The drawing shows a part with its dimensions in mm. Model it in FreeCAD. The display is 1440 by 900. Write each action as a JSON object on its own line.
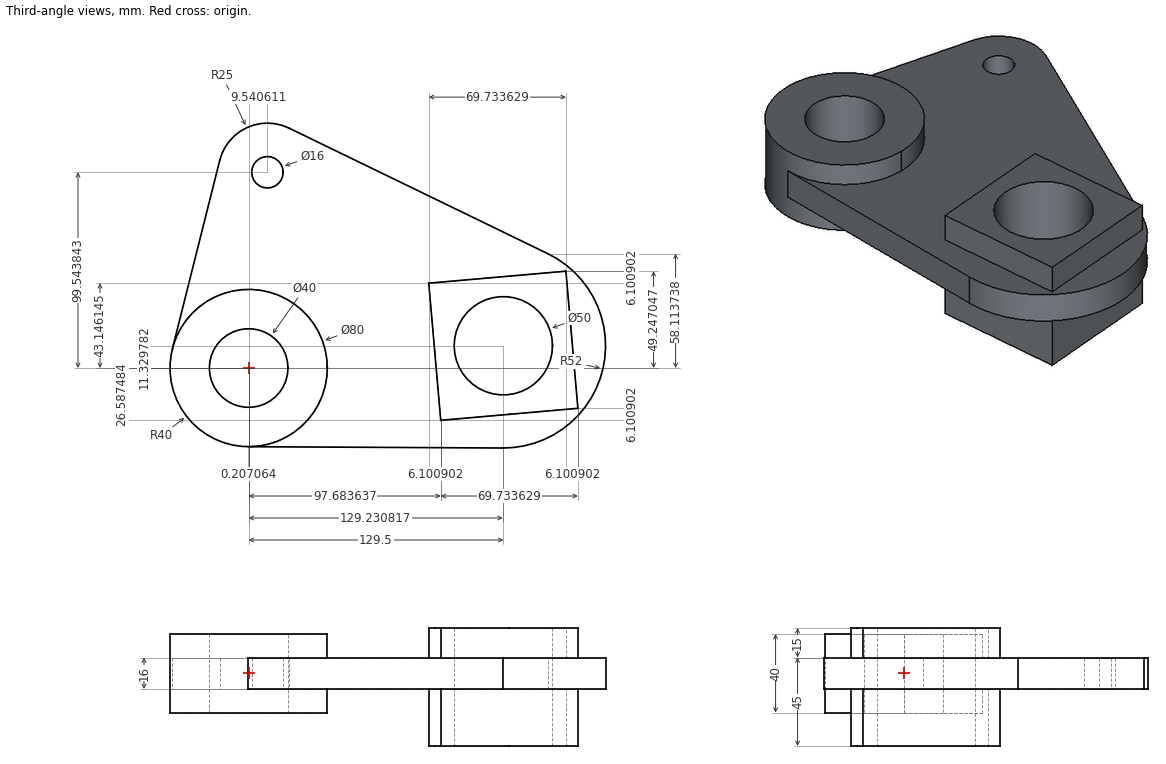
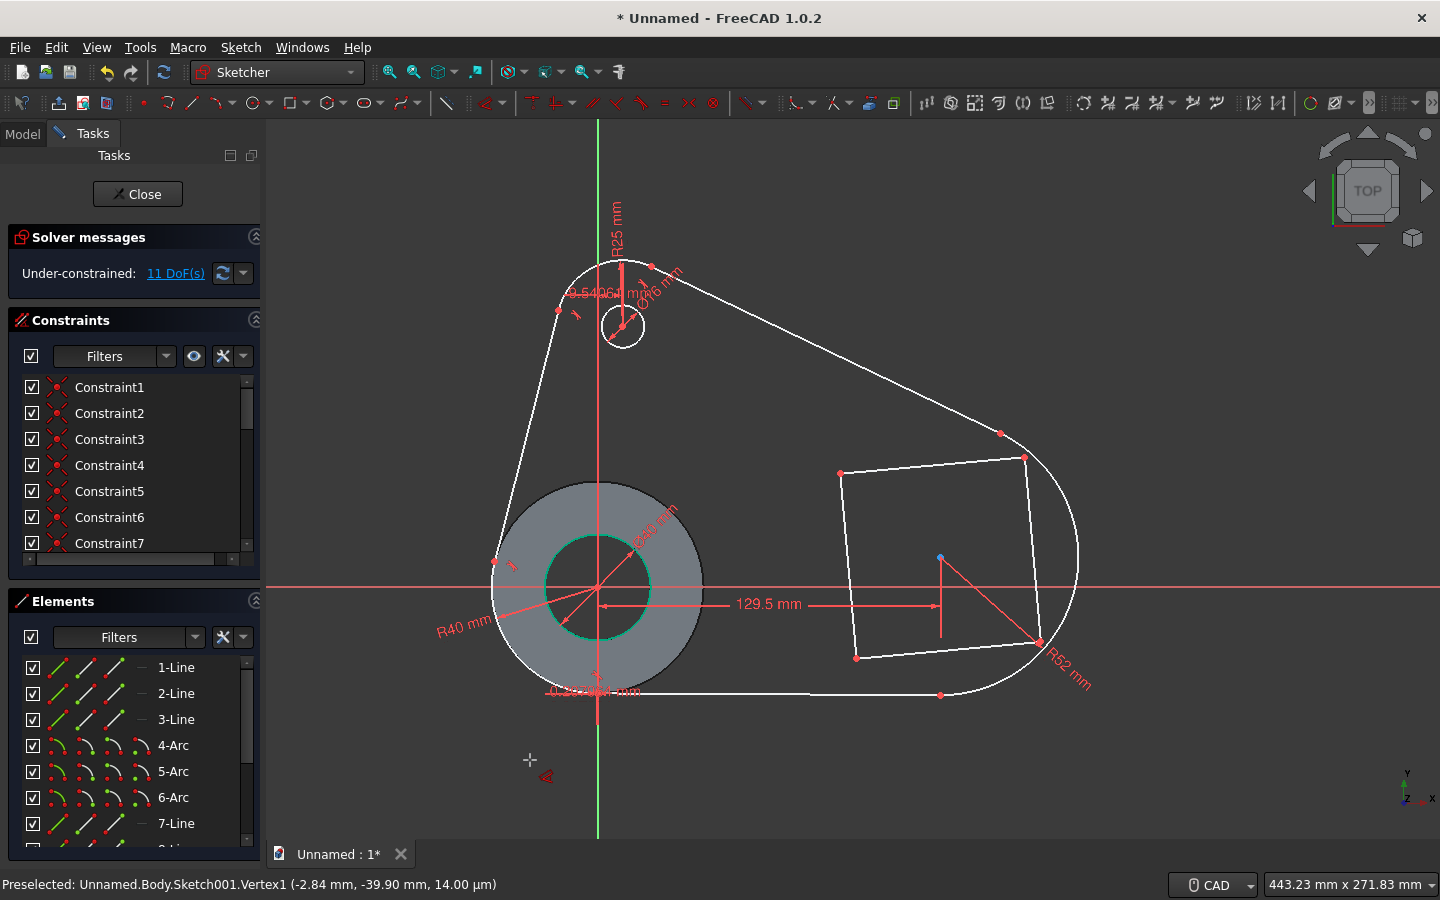
{"action": "scroll", "coordinate": [852, 603], "scroll_direction": "up", "scroll_amount": 5}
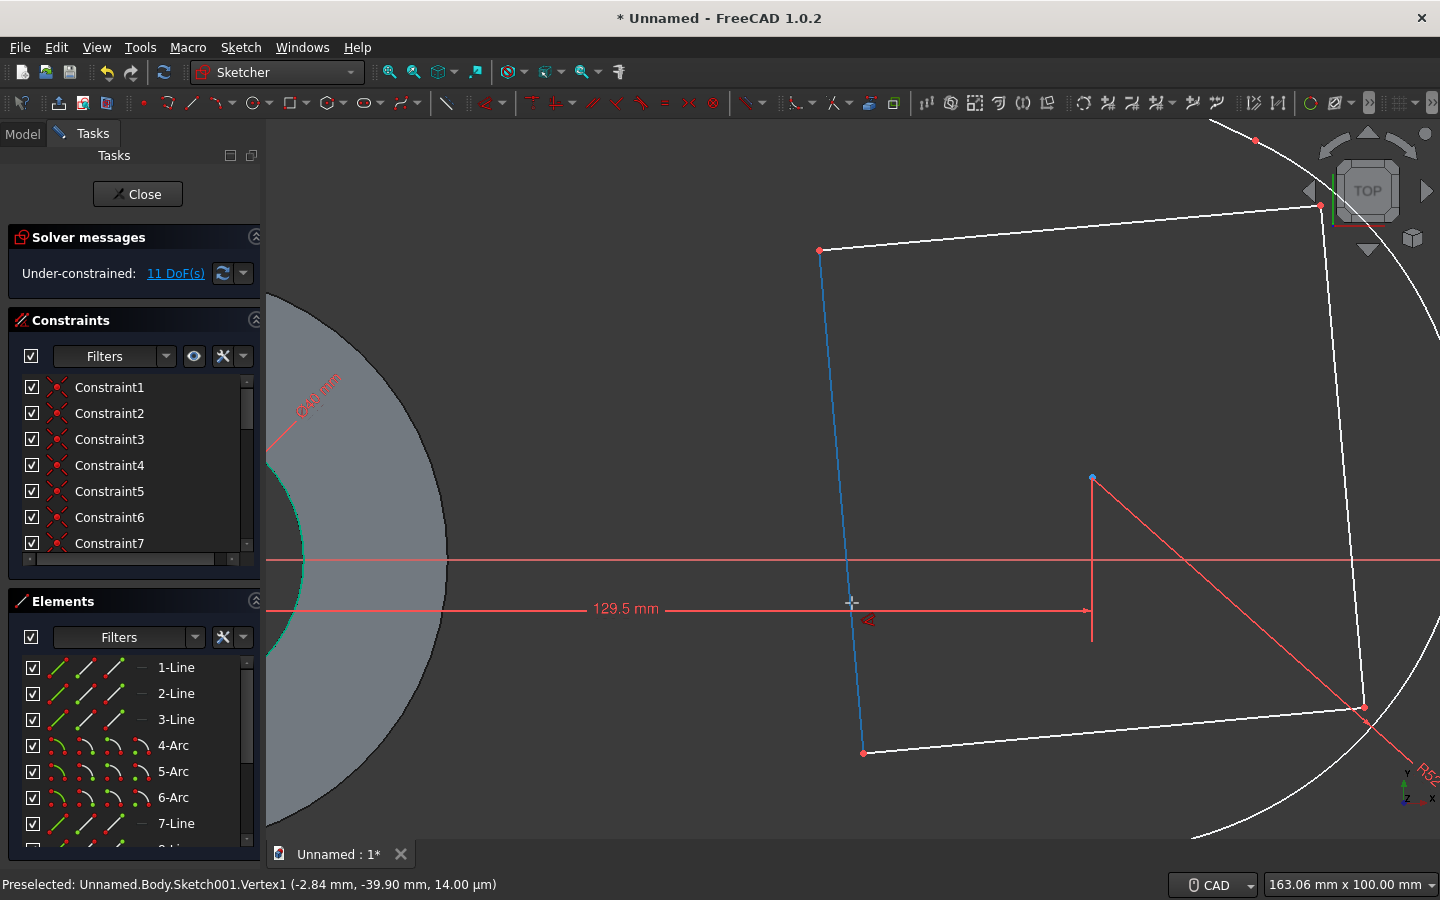
{"action": "left_click", "coordinate": [850, 603]}
{"action": "left_click", "coordinate": [841, 788]}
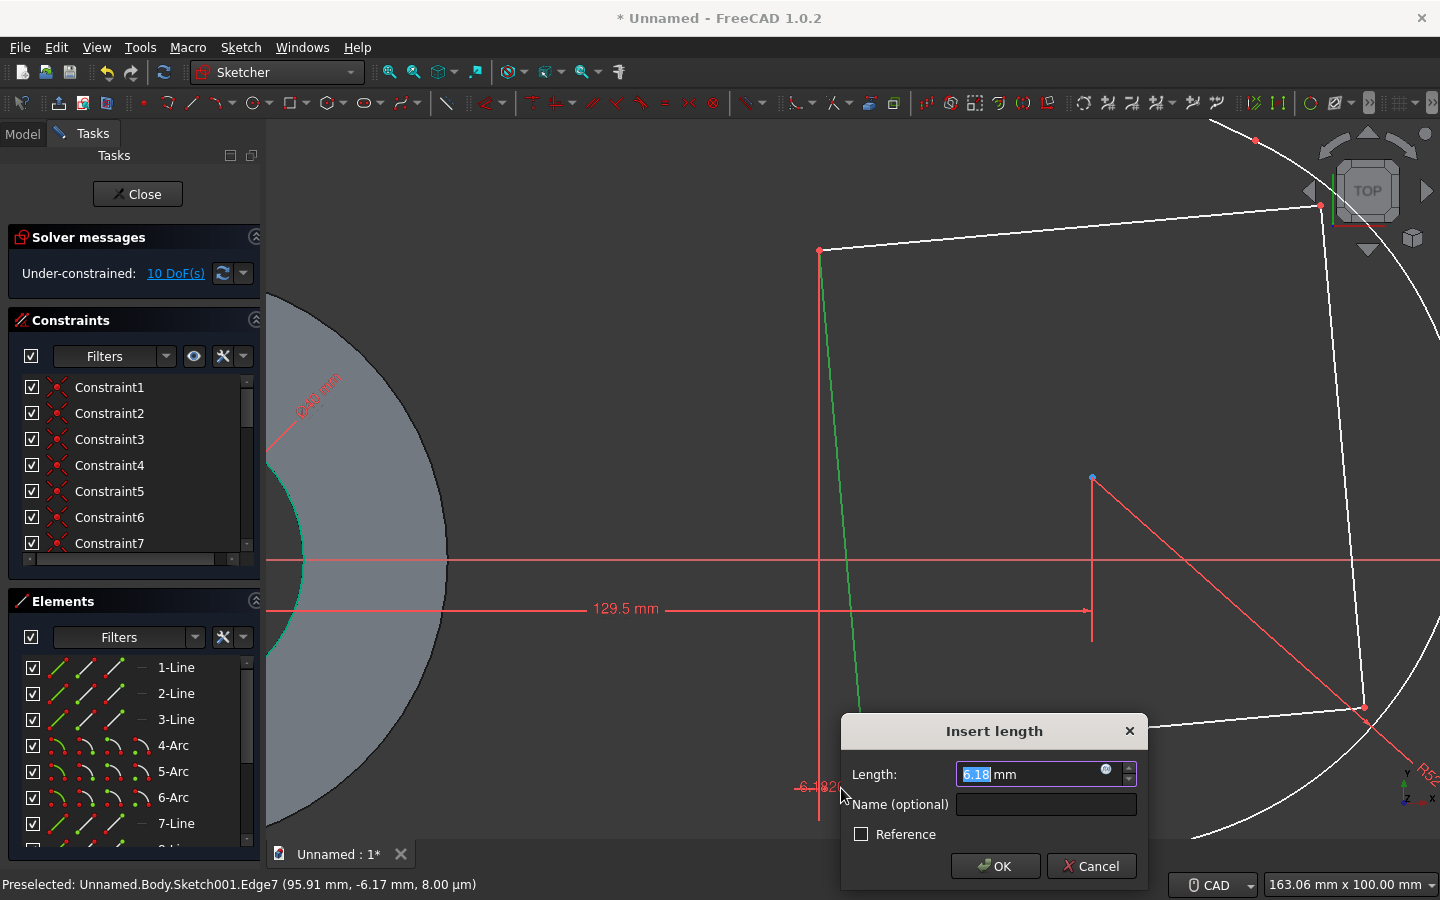
{"action": "type", "text": "6.100902"}
{"action": "key", "text": "Return"}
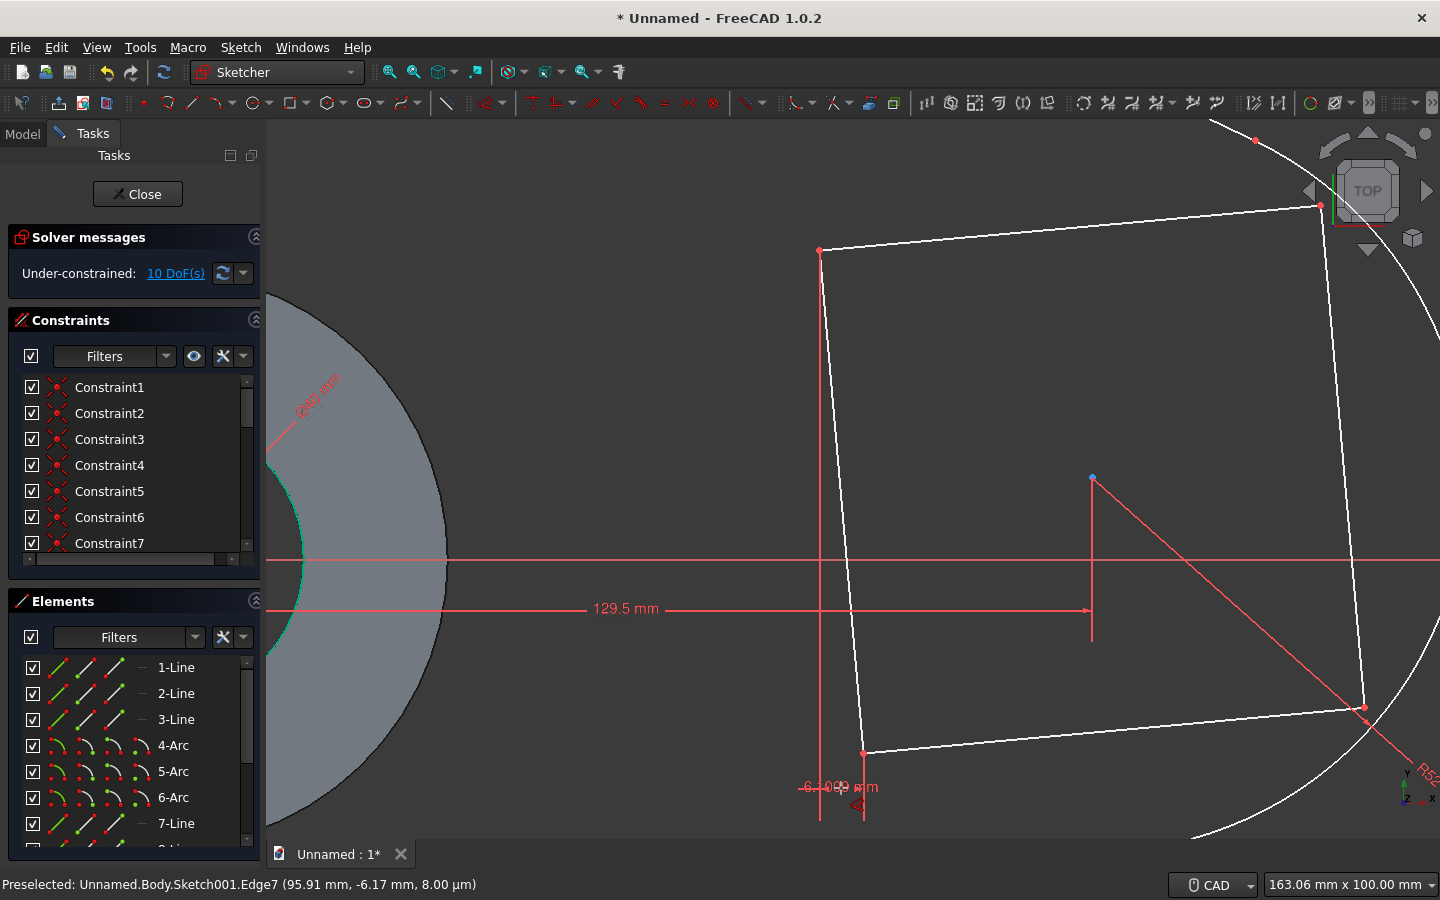
{"action": "left_click", "coordinate": [970, 237]}
{"action": "left_click", "coordinate": [786, 228]}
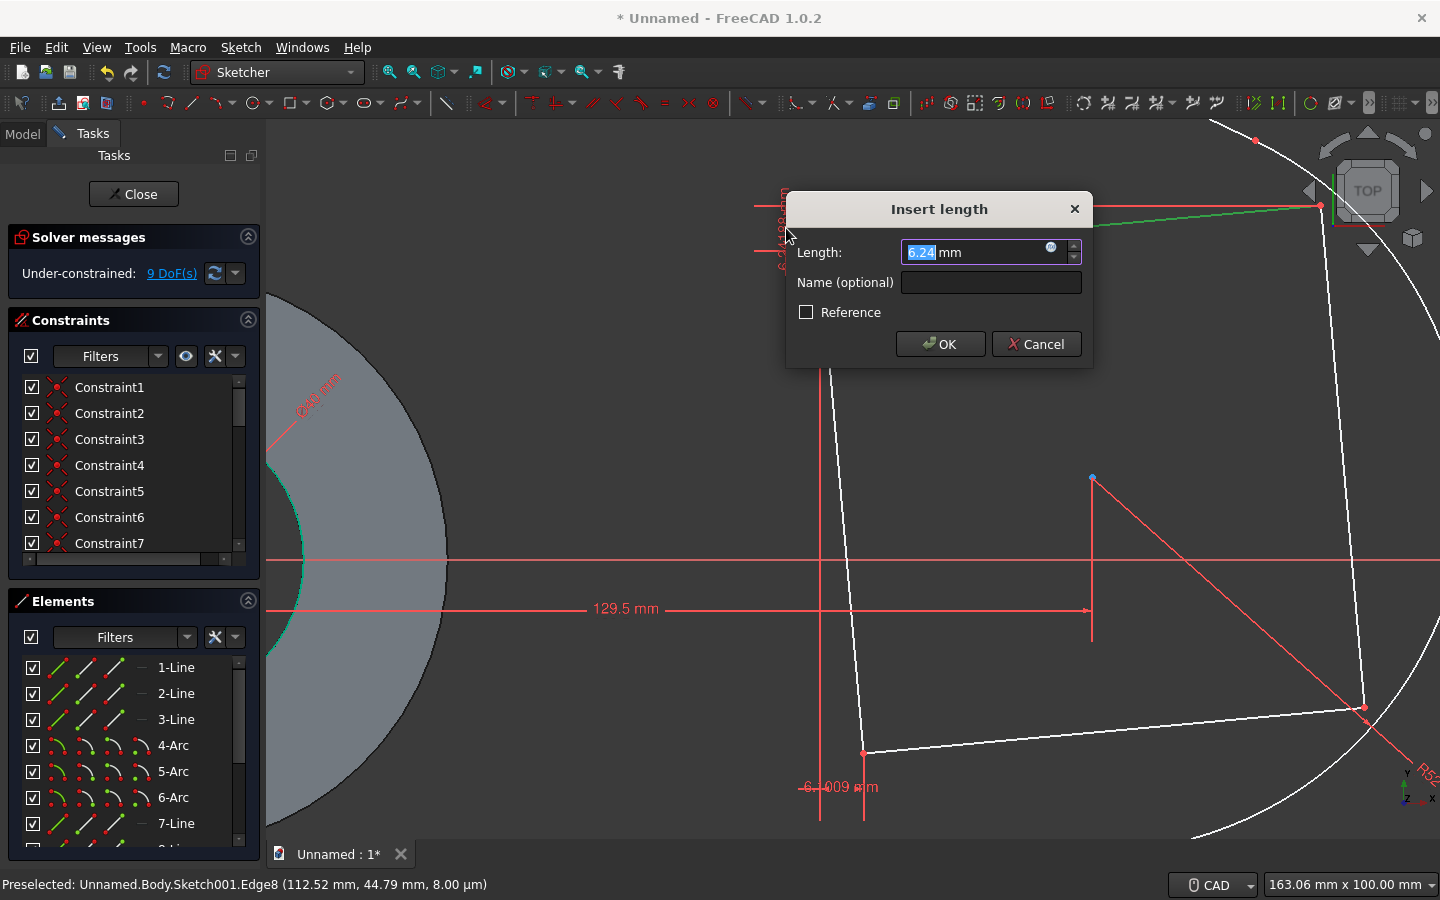
{"action": "type", "text": "6.100902"}
{"action": "key", "text": "Return"}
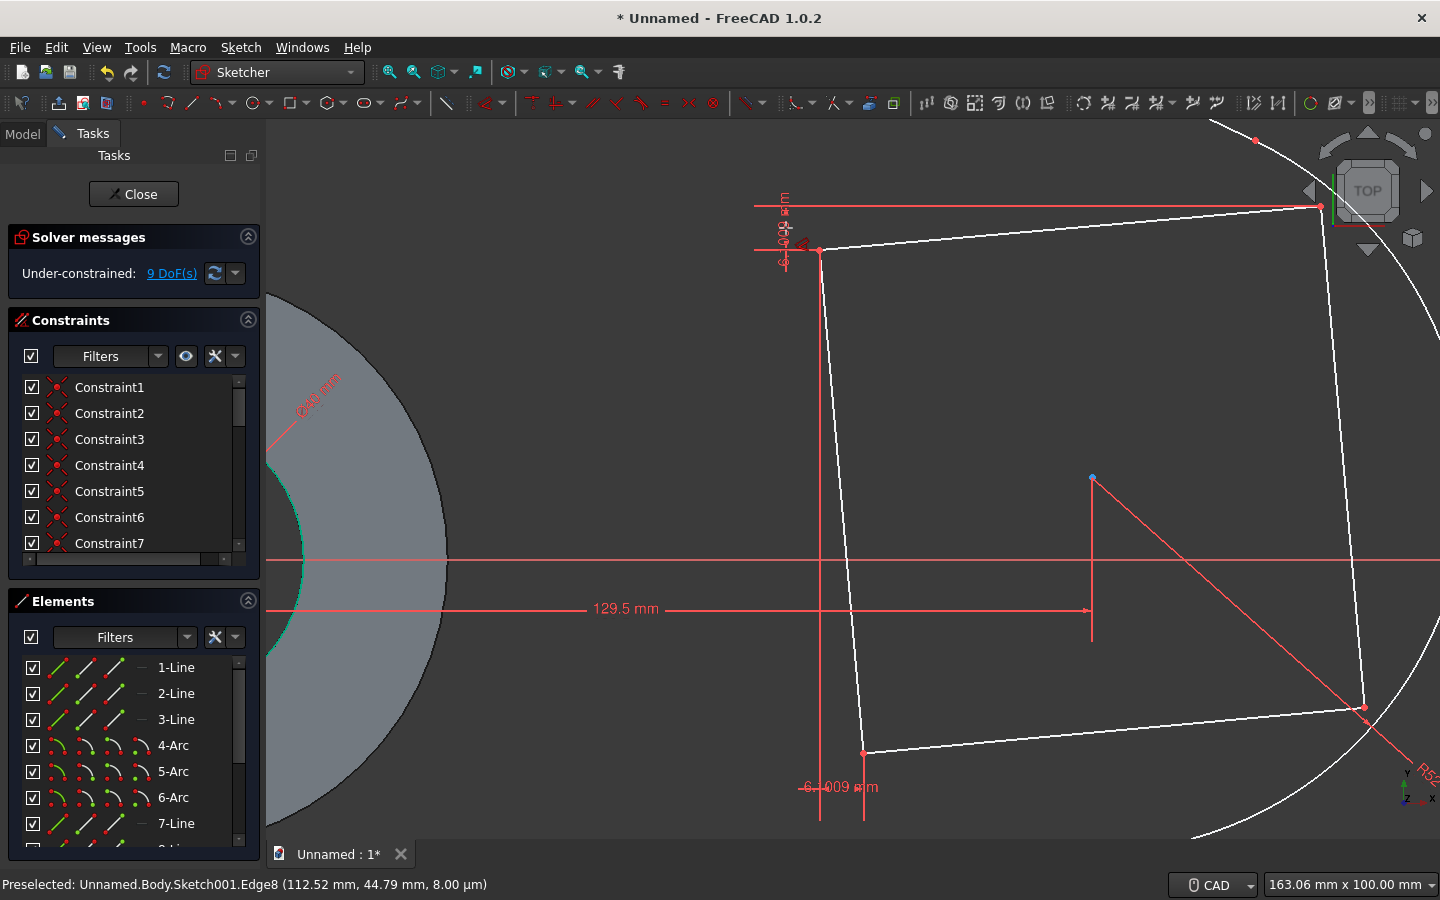
{"action": "scroll", "coordinate": [852, 603], "scroll_direction": "down", "scroll_amount": 5}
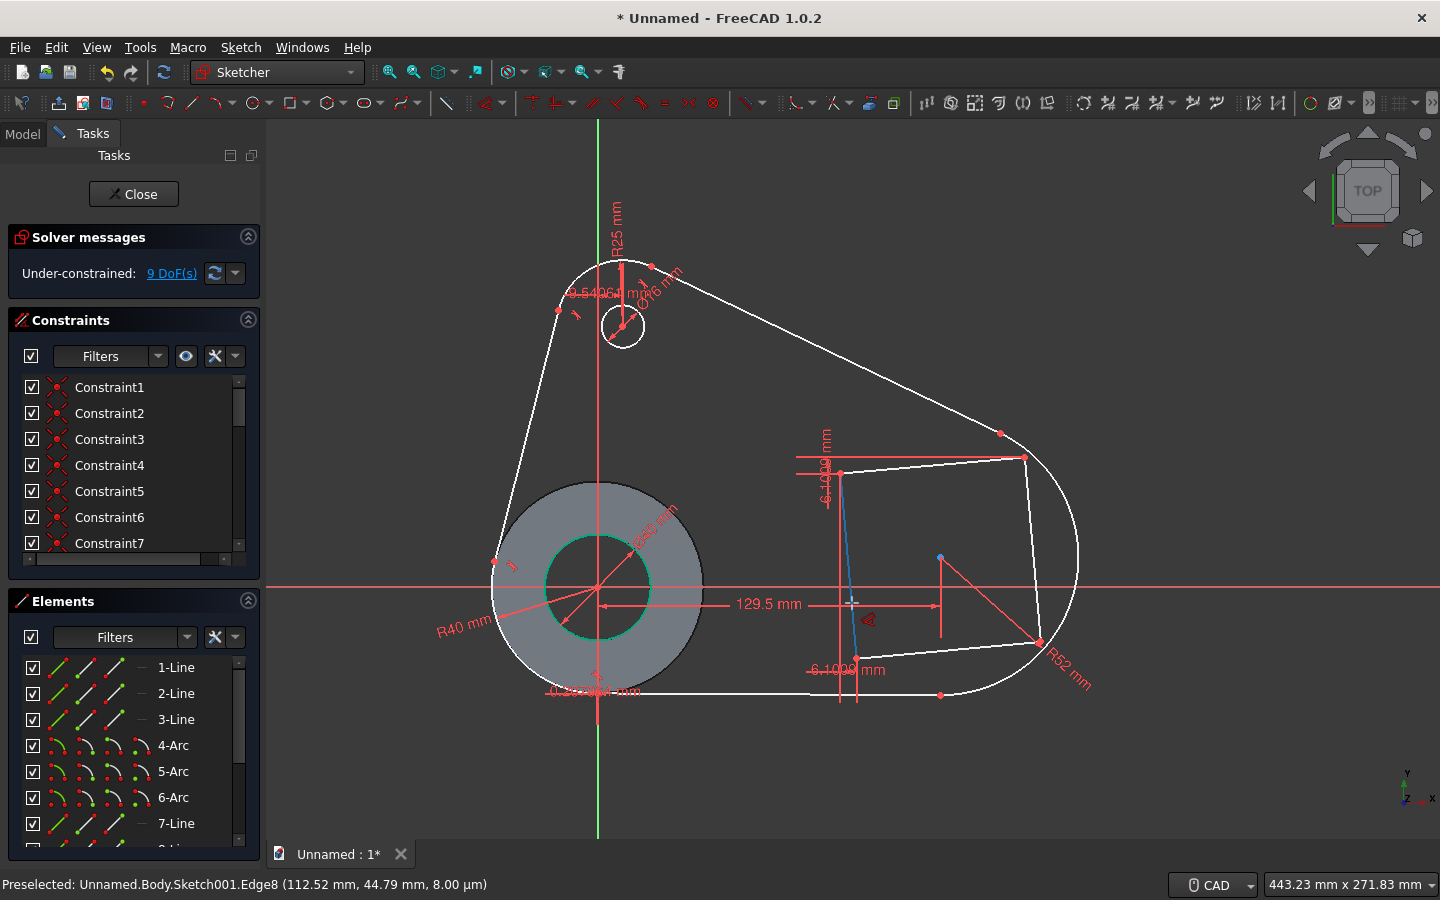
{"action": "scroll", "coordinate": [1030, 513], "scroll_direction": "up", "scroll_amount": 5}